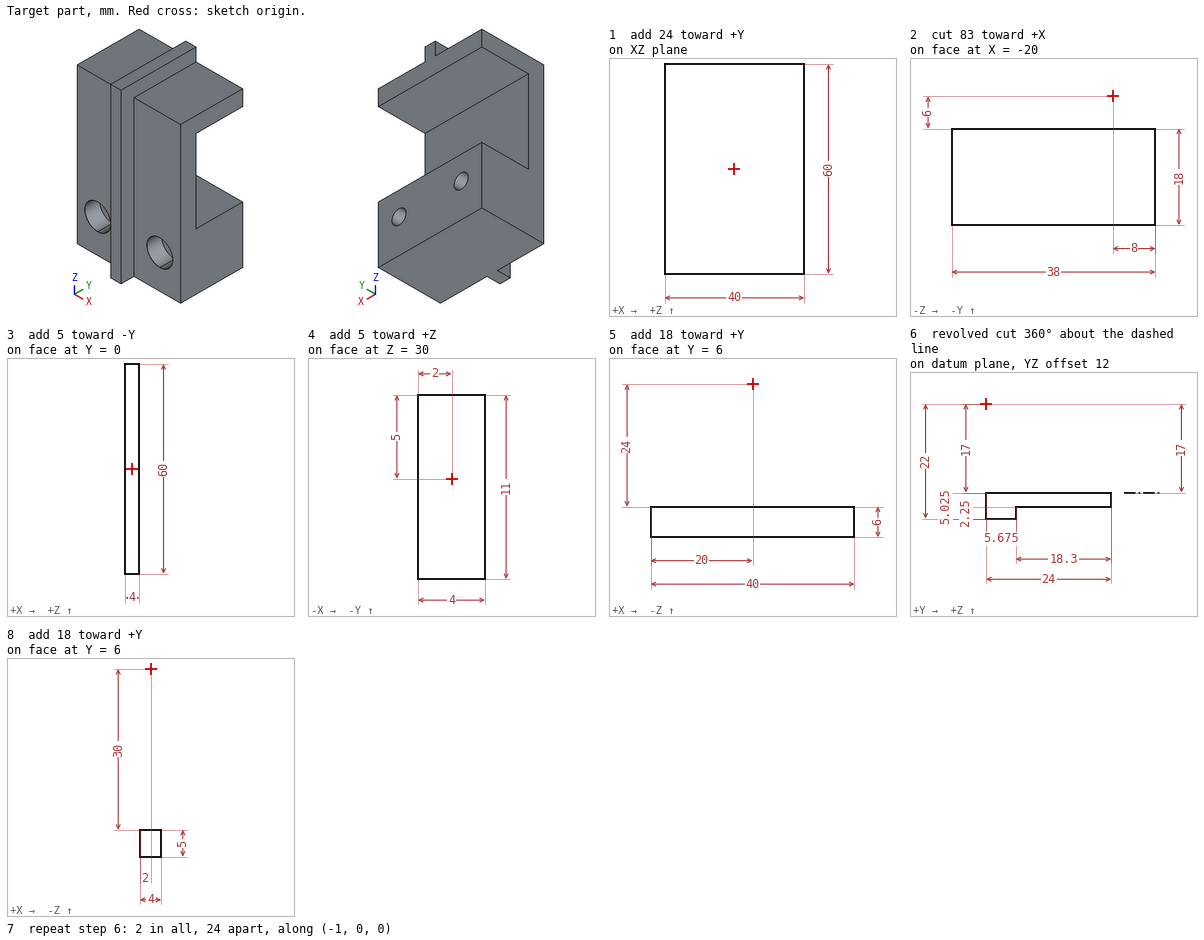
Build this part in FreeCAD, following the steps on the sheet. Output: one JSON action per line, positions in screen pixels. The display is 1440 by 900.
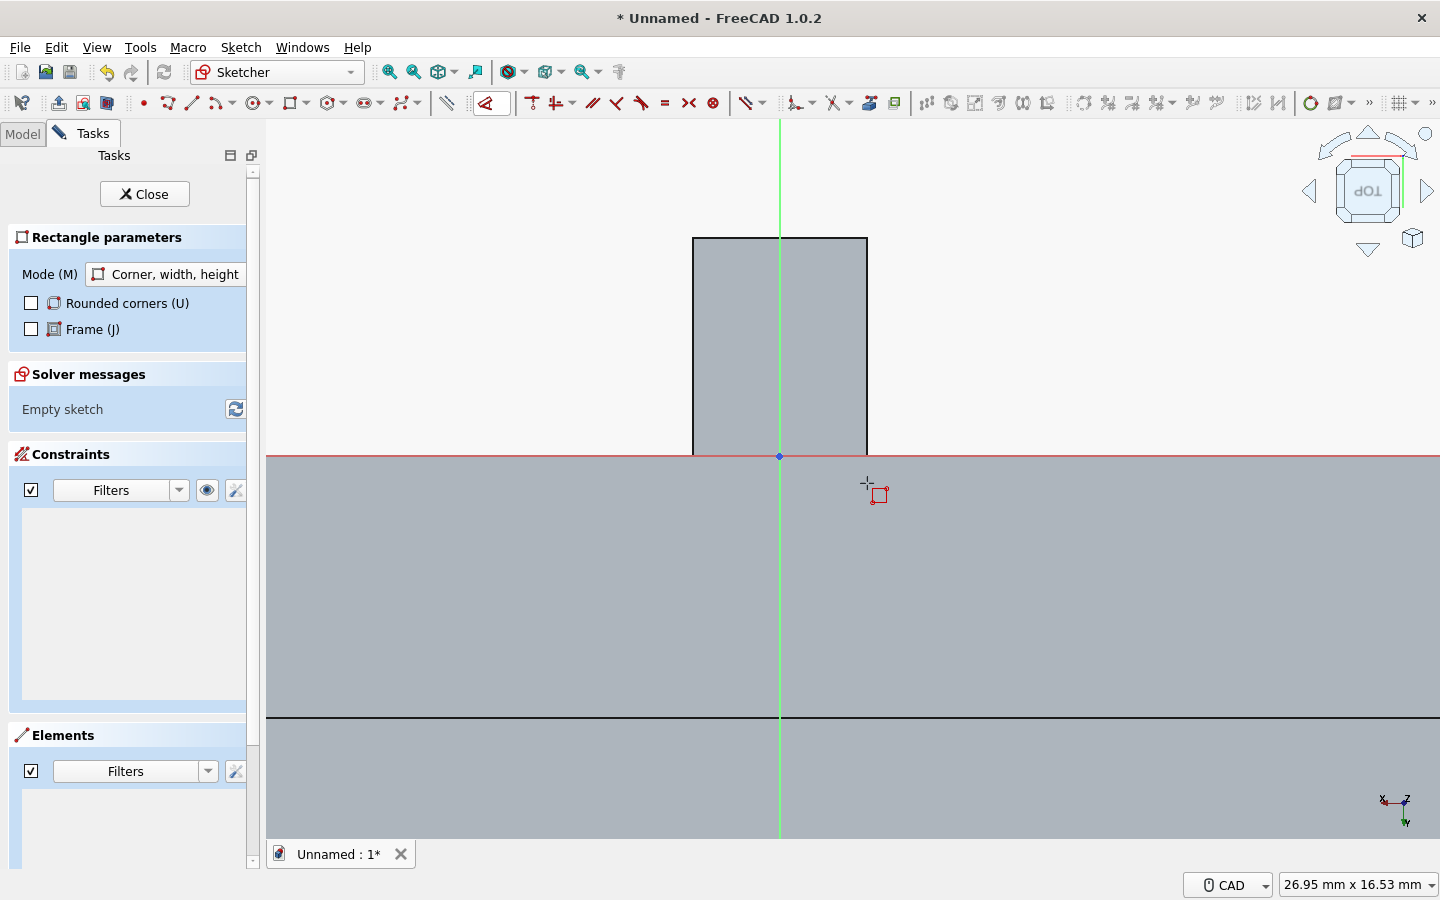
{"action": "left_click", "coordinate": [693, 238]}
{"action": "mouse_move", "coordinate": [867, 718]}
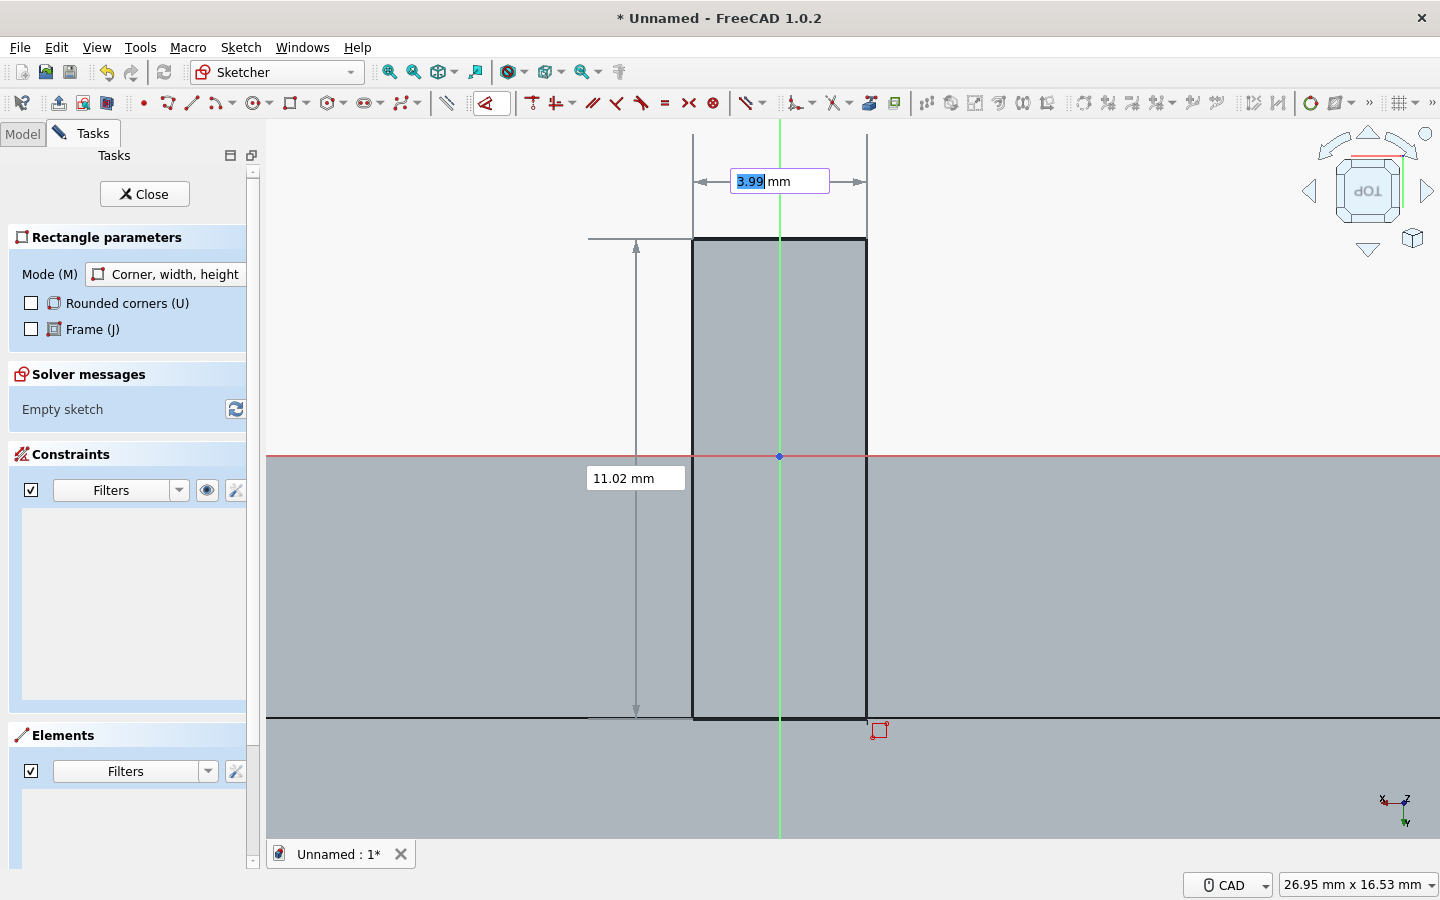
{"action": "type", "text": "4"}
{"action": "key", "text": "Tab"}
{"action": "type", "text": "11"}
{"action": "key", "text": "Return"}
{"action": "key", "text": "Escape"}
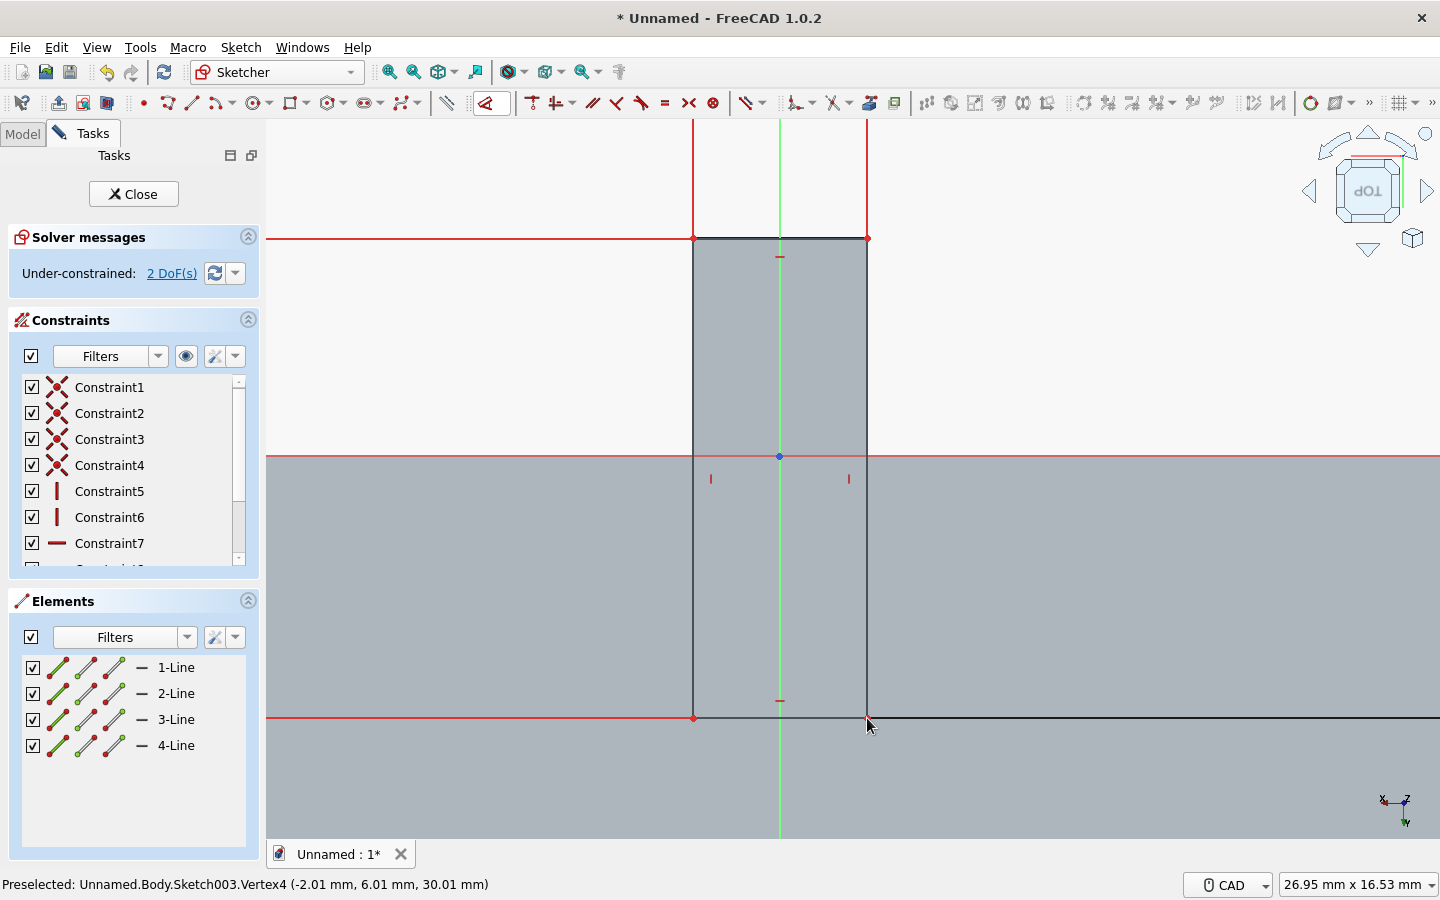
{"action": "key", "text": "d"}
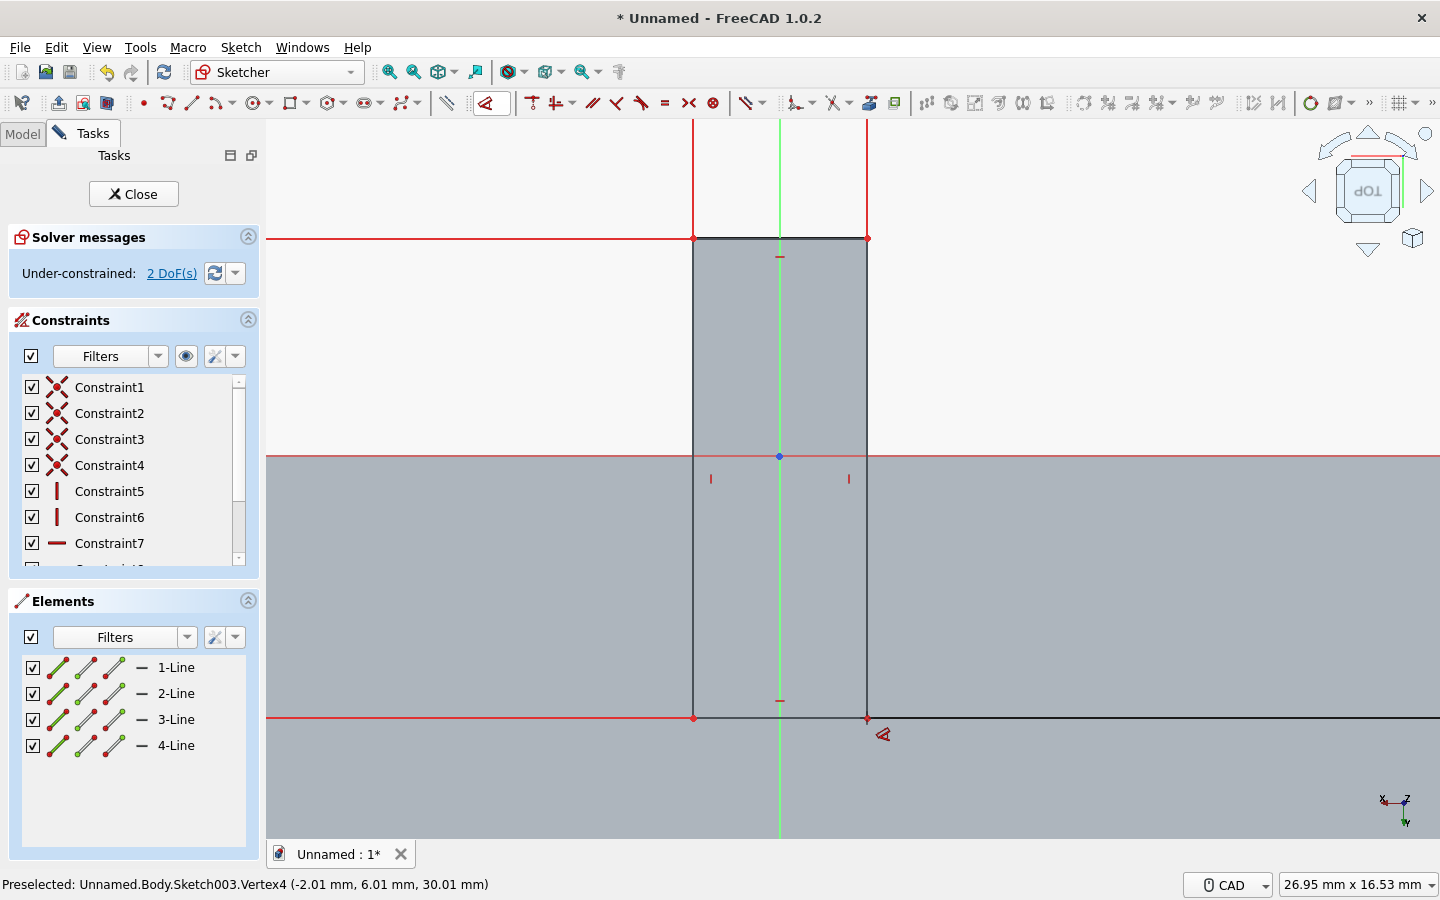
{"action": "left_click", "coordinate": [693, 239]}
{"action": "left_click", "coordinate": [736, 205]}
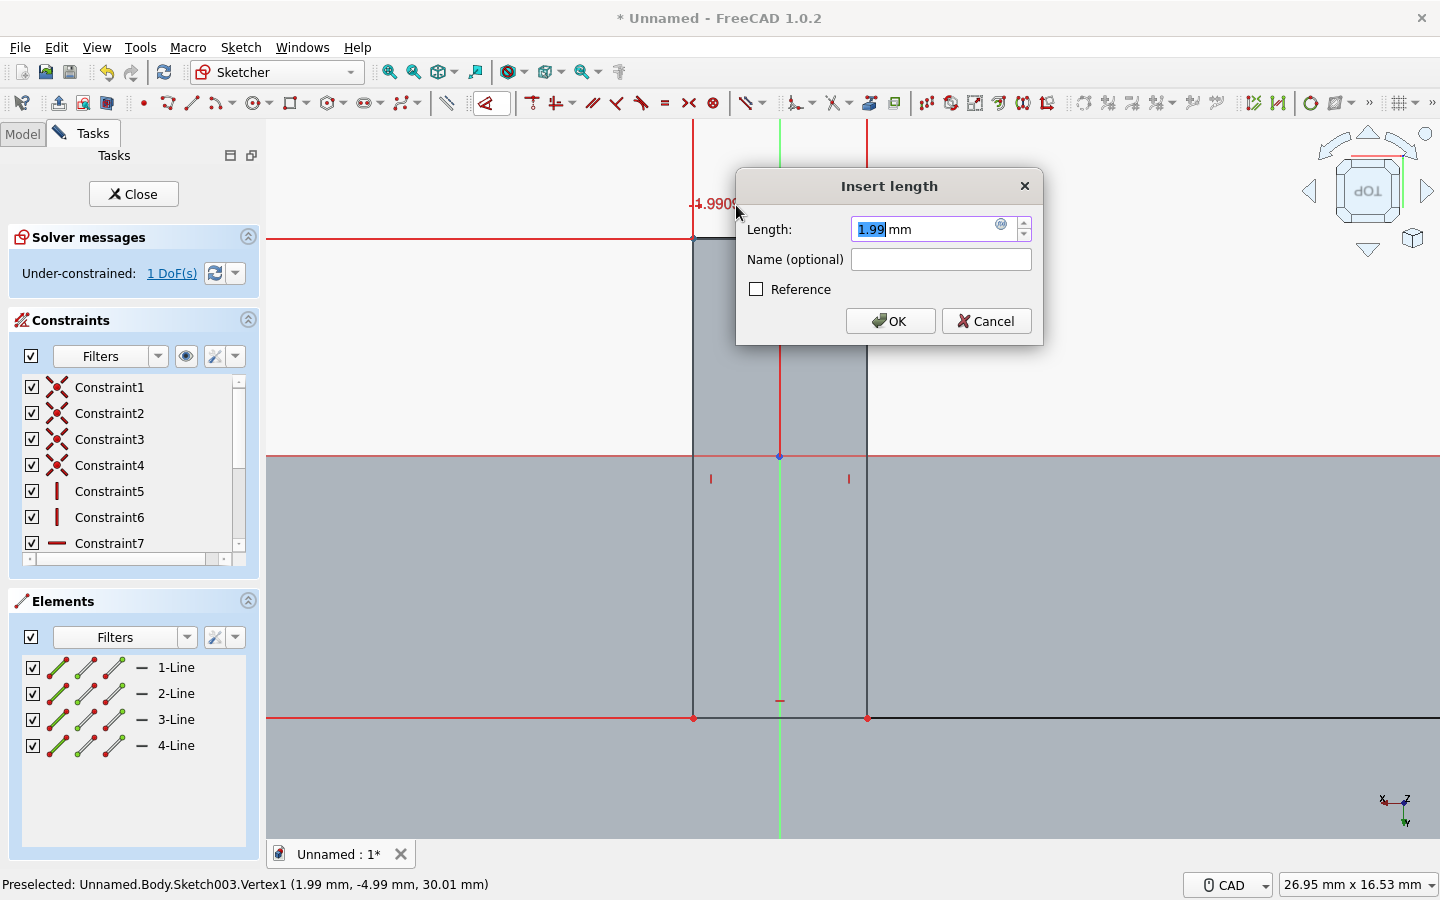
{"action": "type", "text": "2"}
{"action": "key", "text": "Return"}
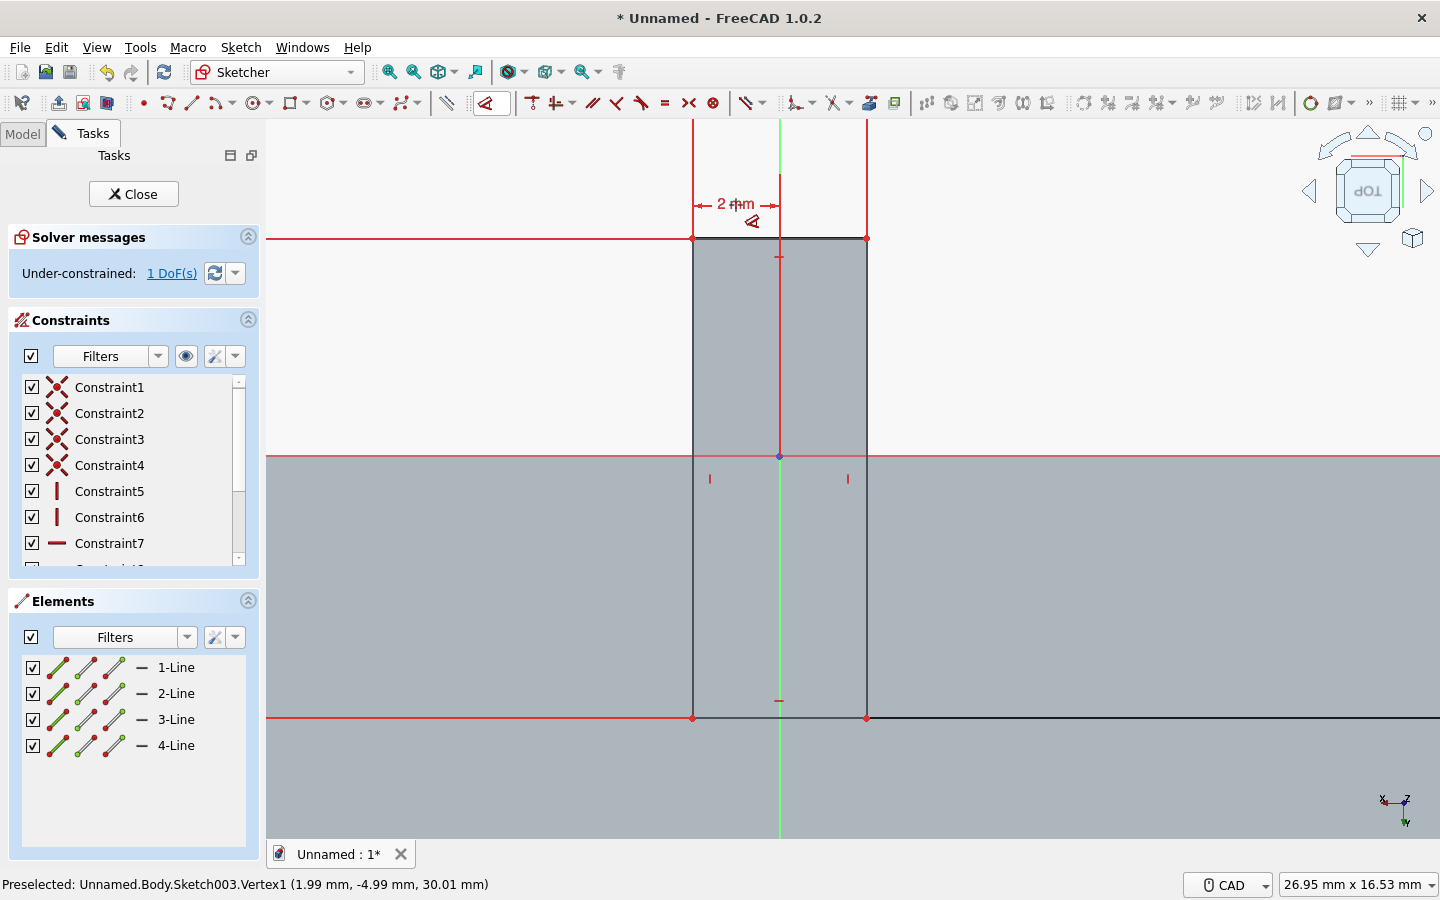
{"action": "left_click", "coordinate": [693, 239]}
{"action": "left_click", "coordinate": [659, 348]}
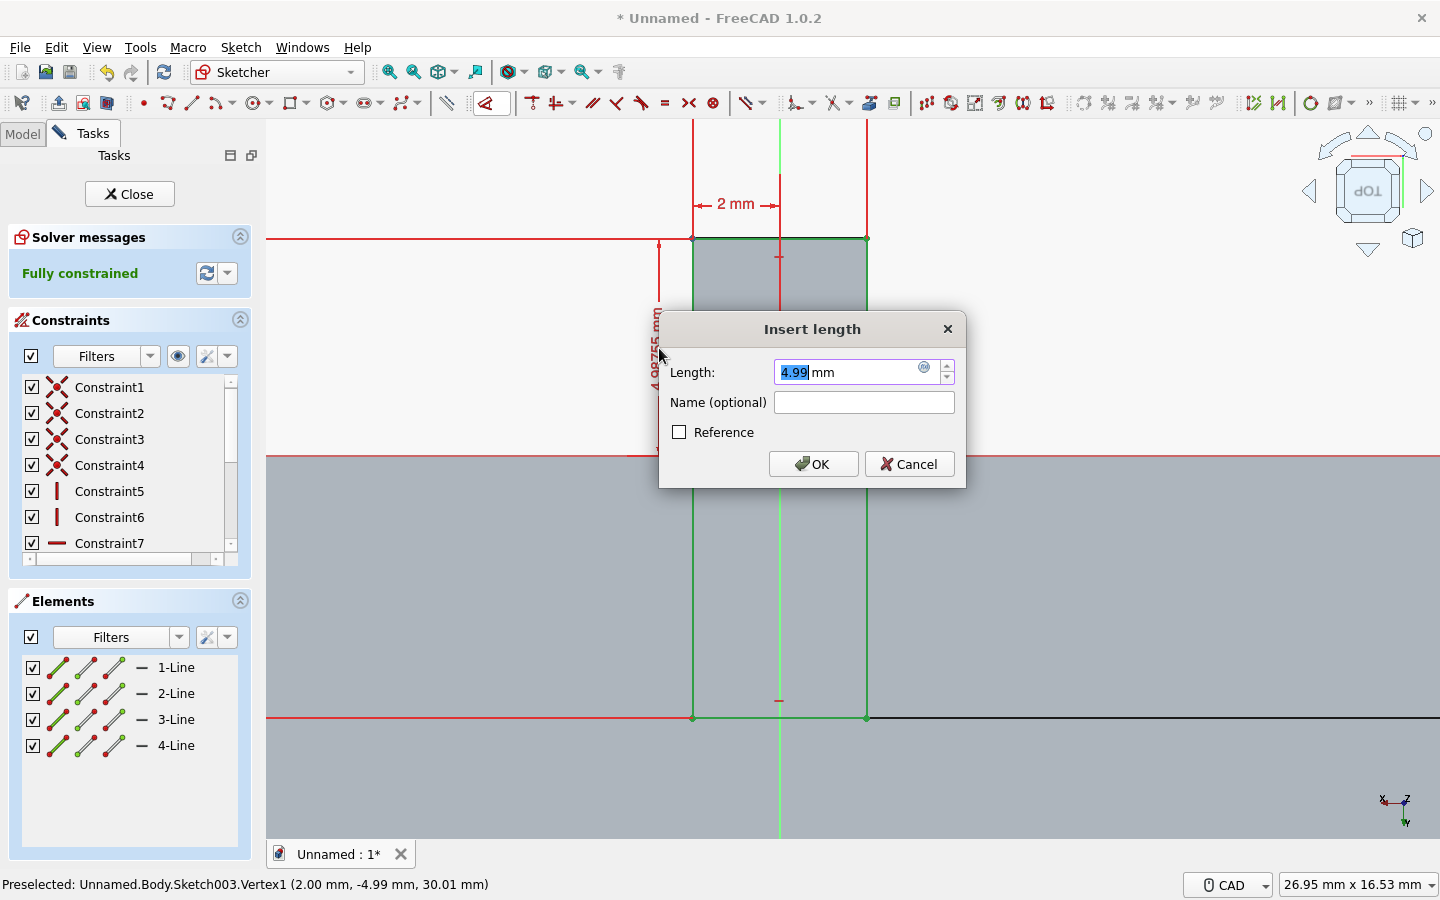
{"action": "type", "text": "5"}
{"action": "key", "text": "Return"}
{"action": "key", "text": "Escape"}